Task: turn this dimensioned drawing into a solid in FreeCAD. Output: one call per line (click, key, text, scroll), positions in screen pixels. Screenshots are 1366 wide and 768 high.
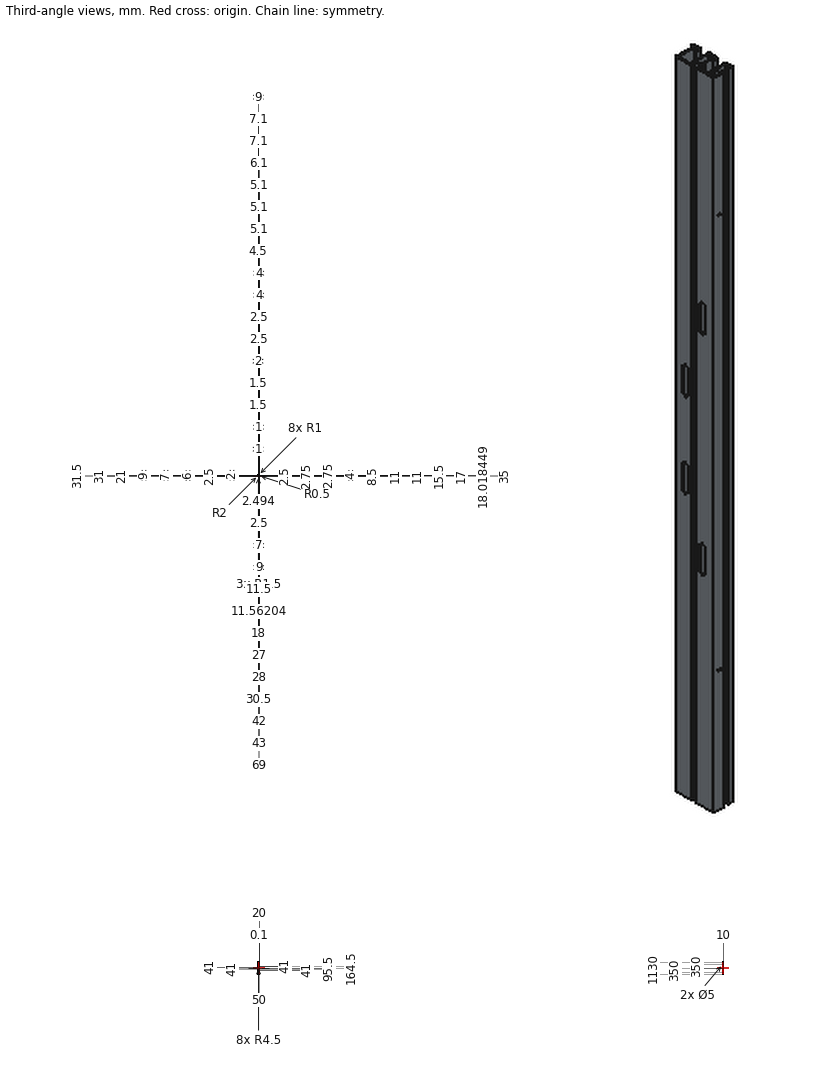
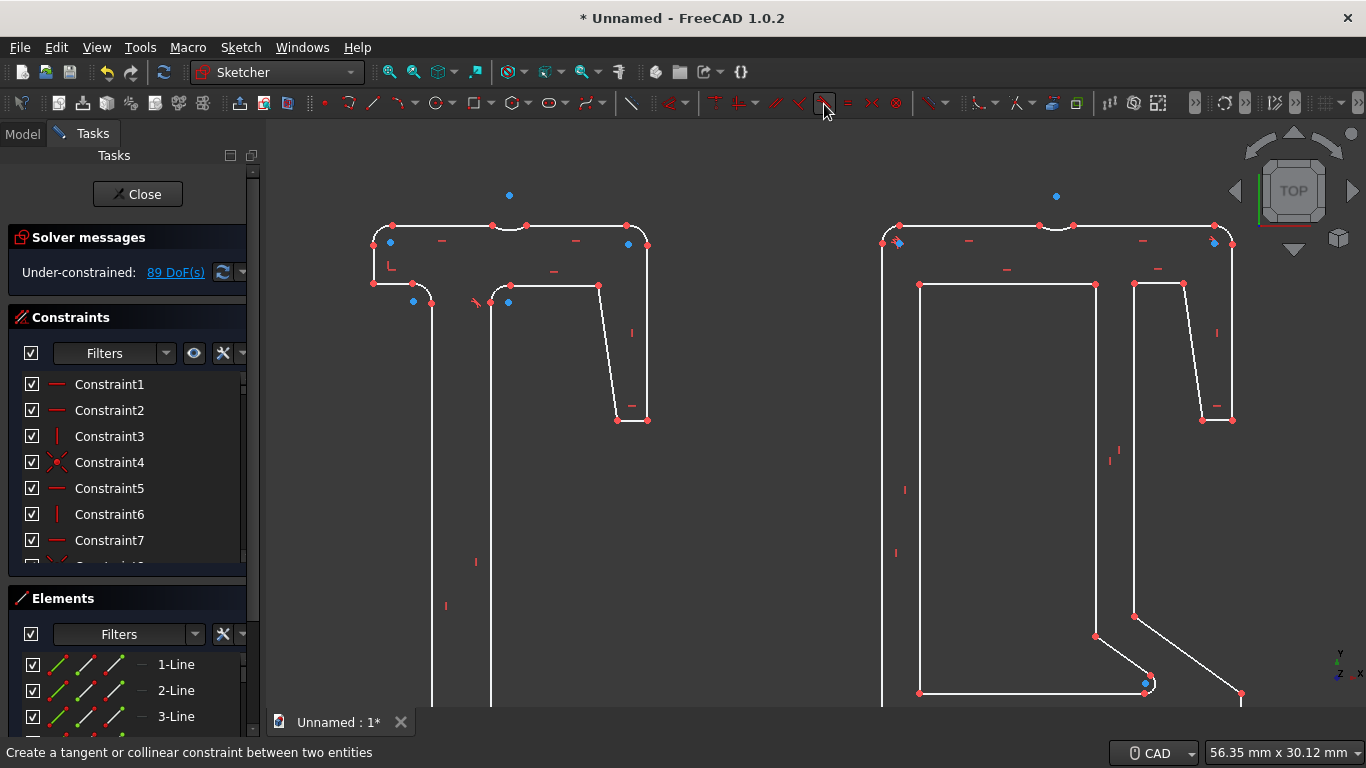
click(537, 286)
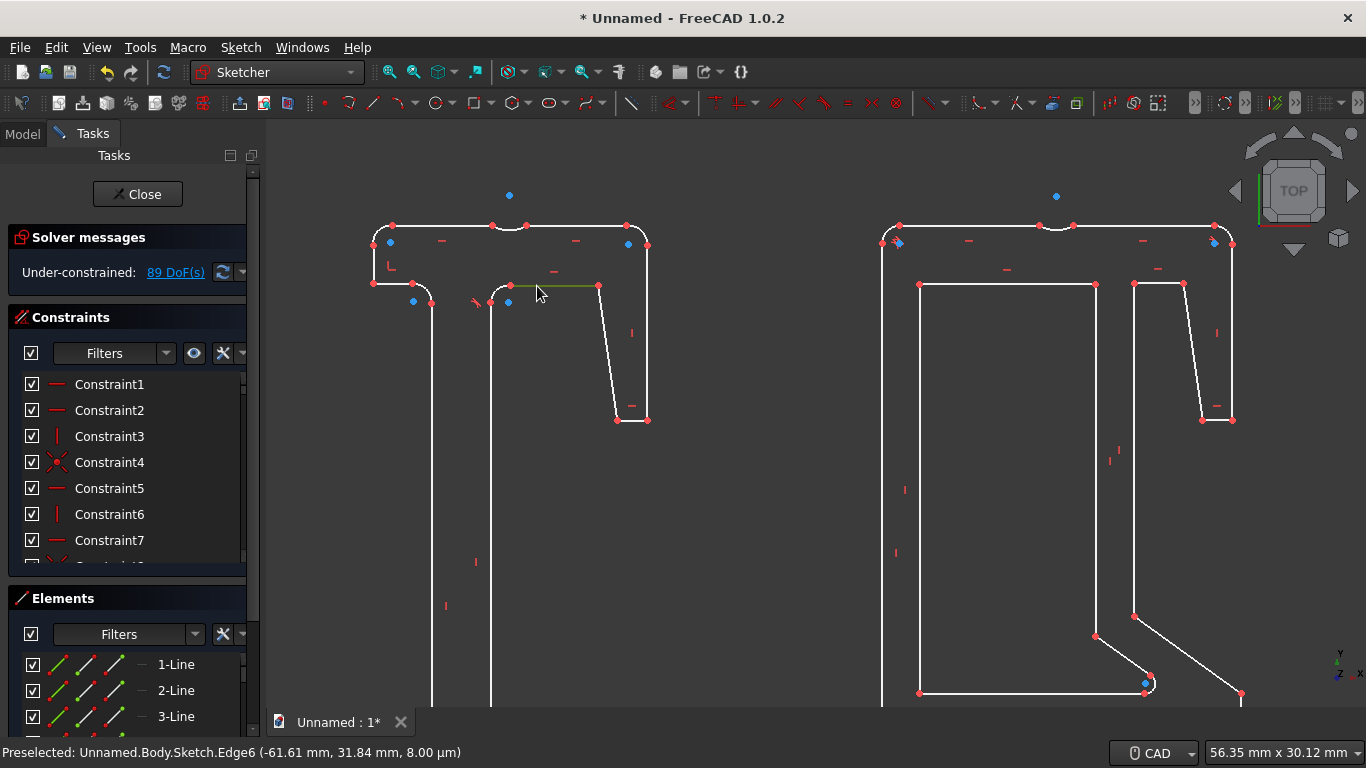
click(497, 290)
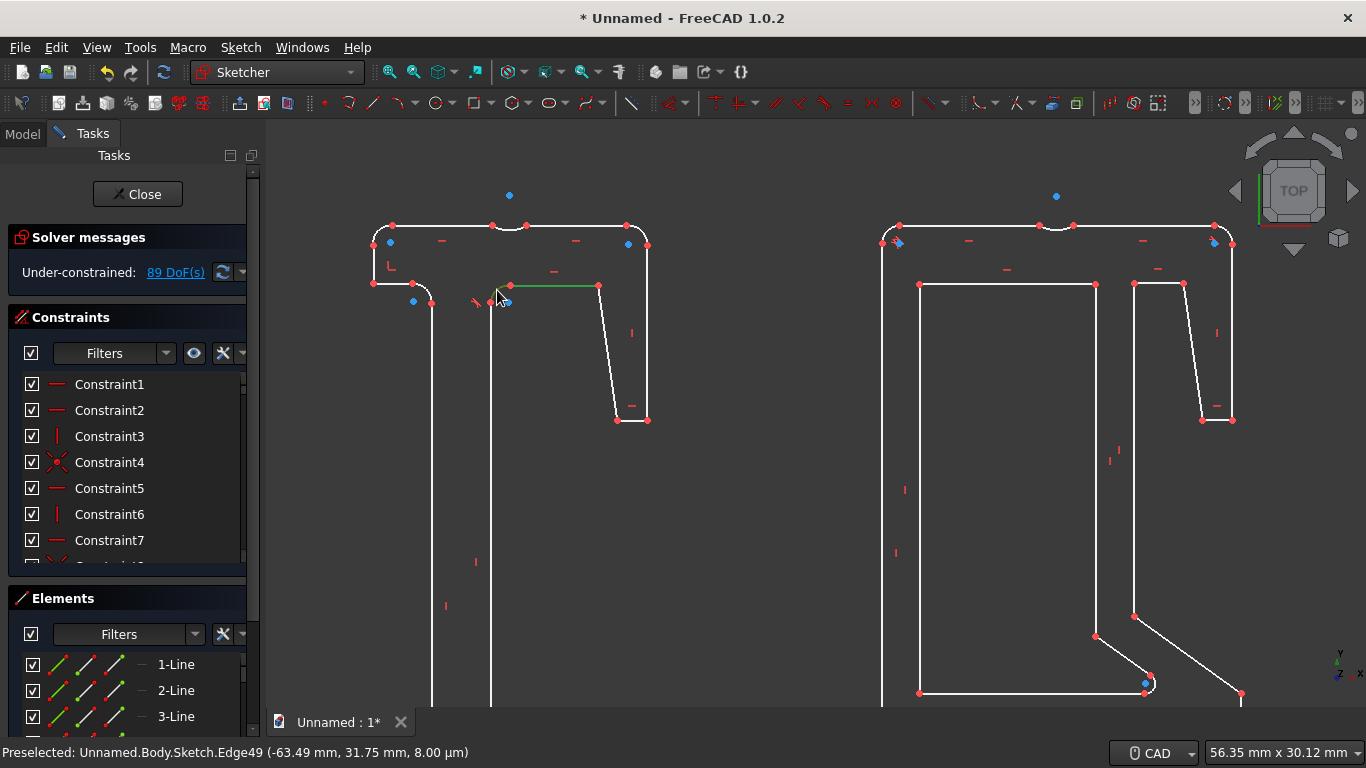
click(824, 104)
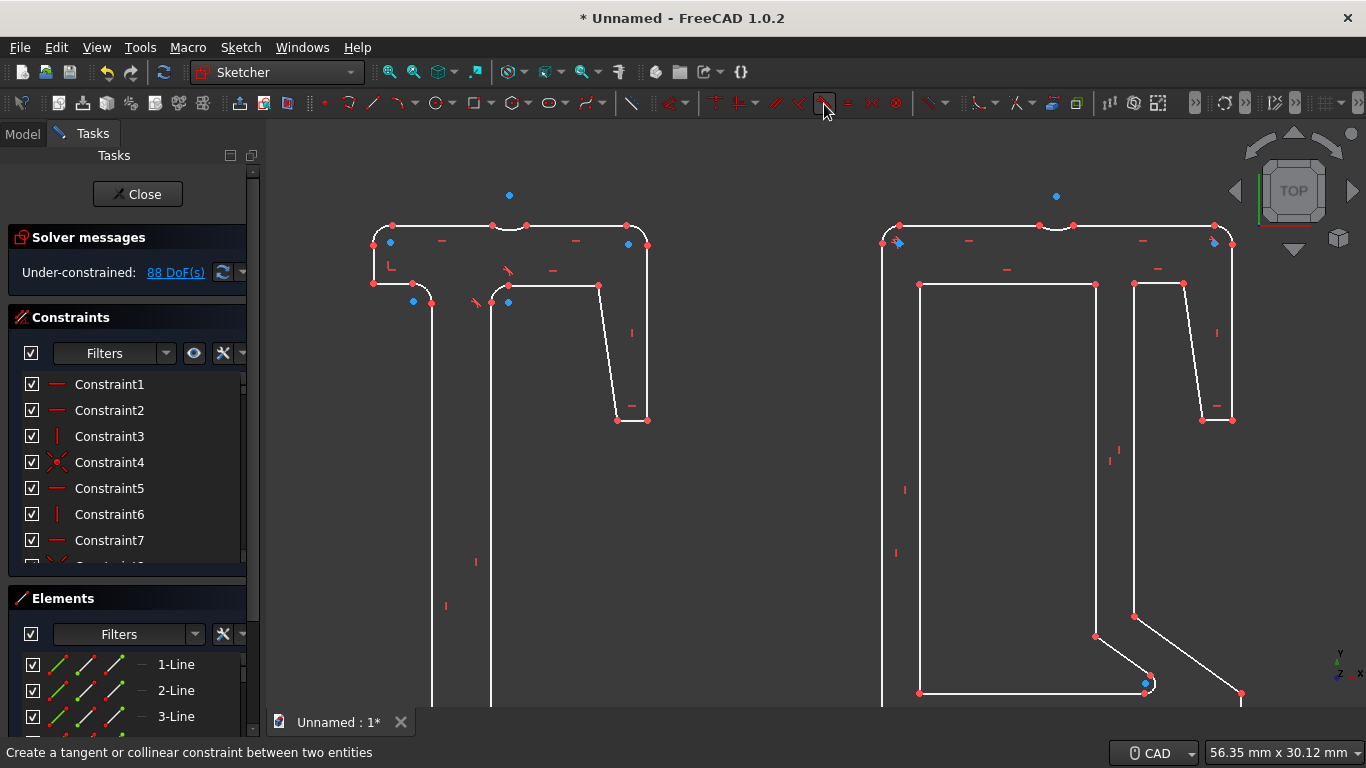
click(647, 368)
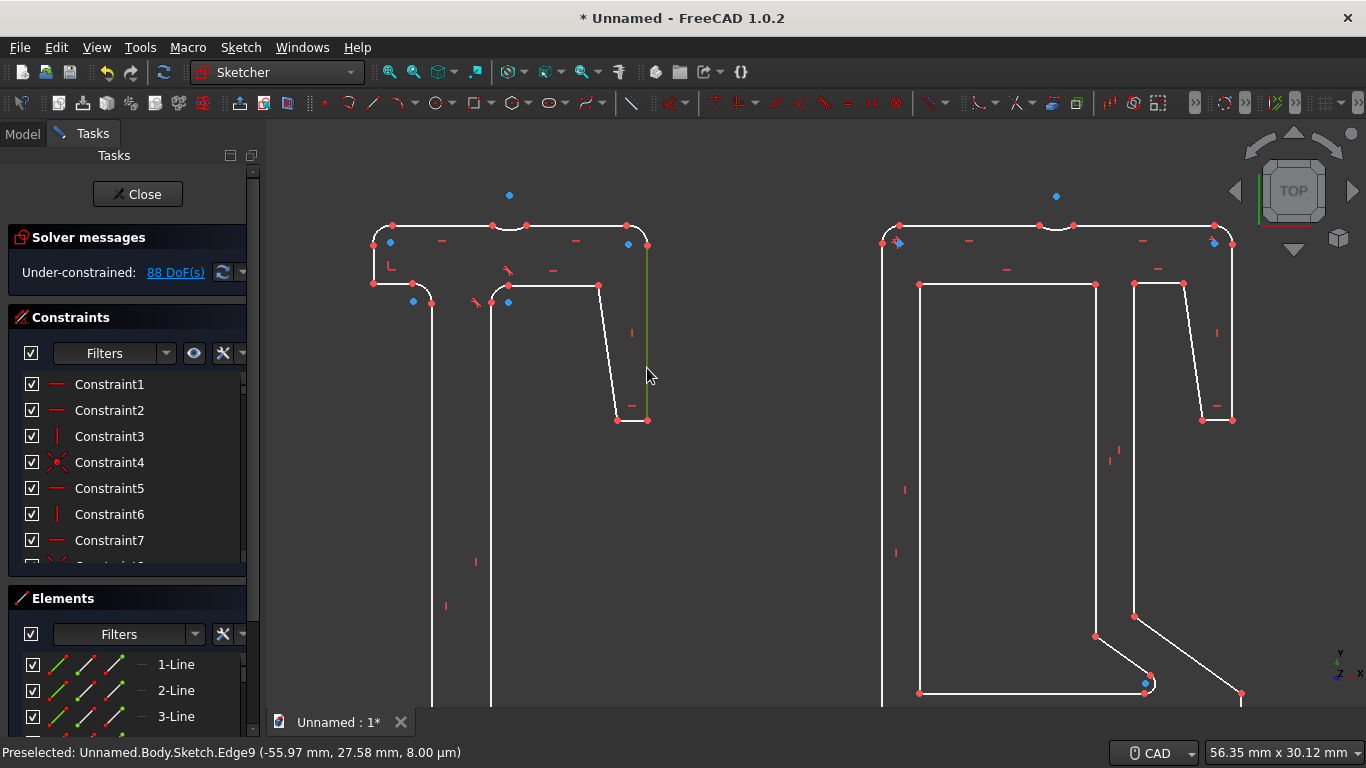
scroll(645, 236, up, 2)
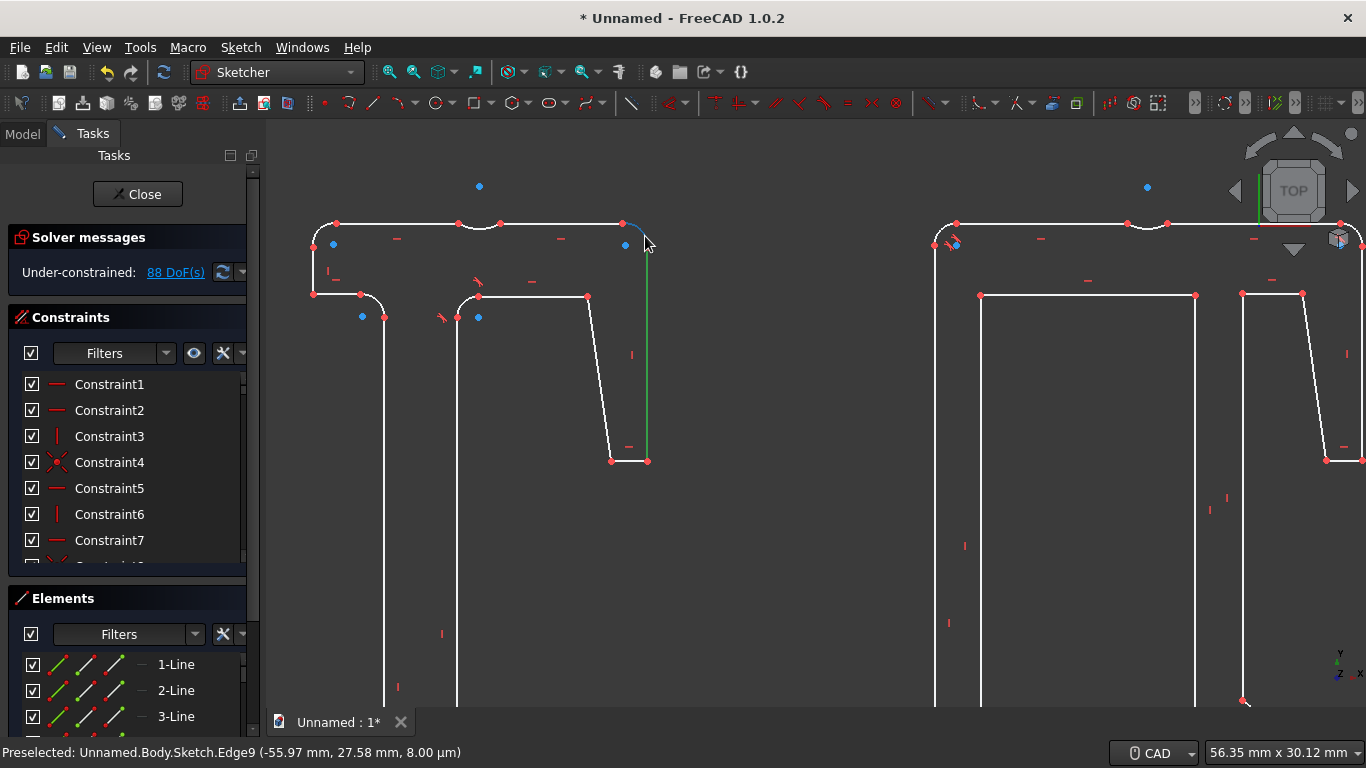
click(645, 236)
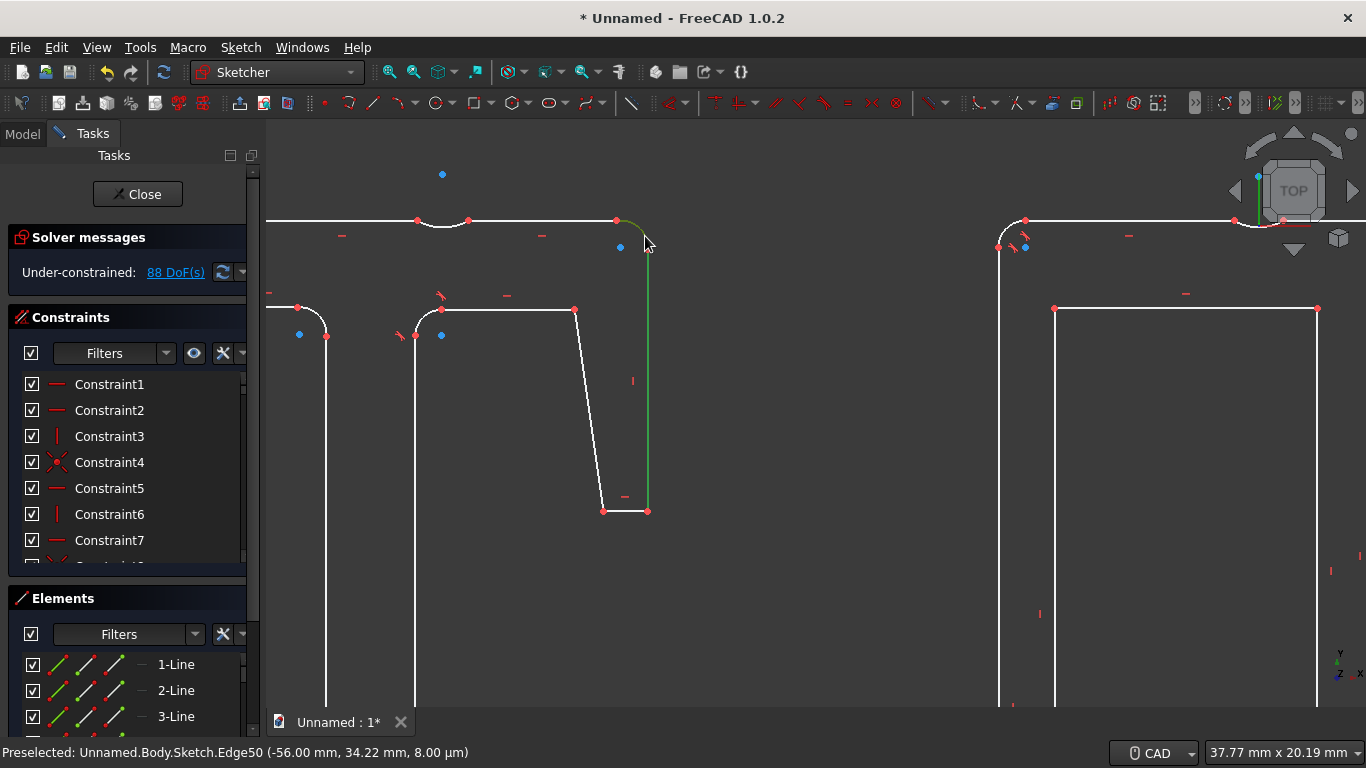
click(824, 104)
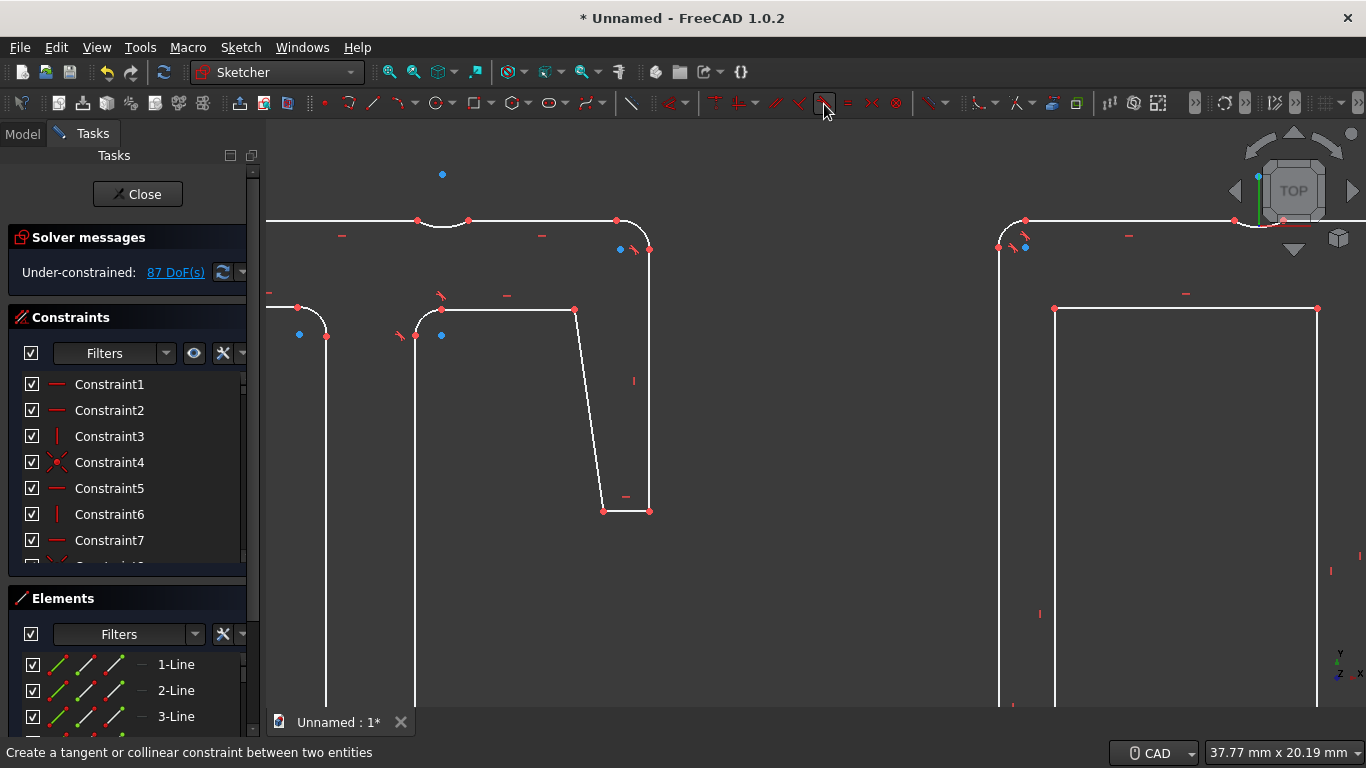
click(572, 221)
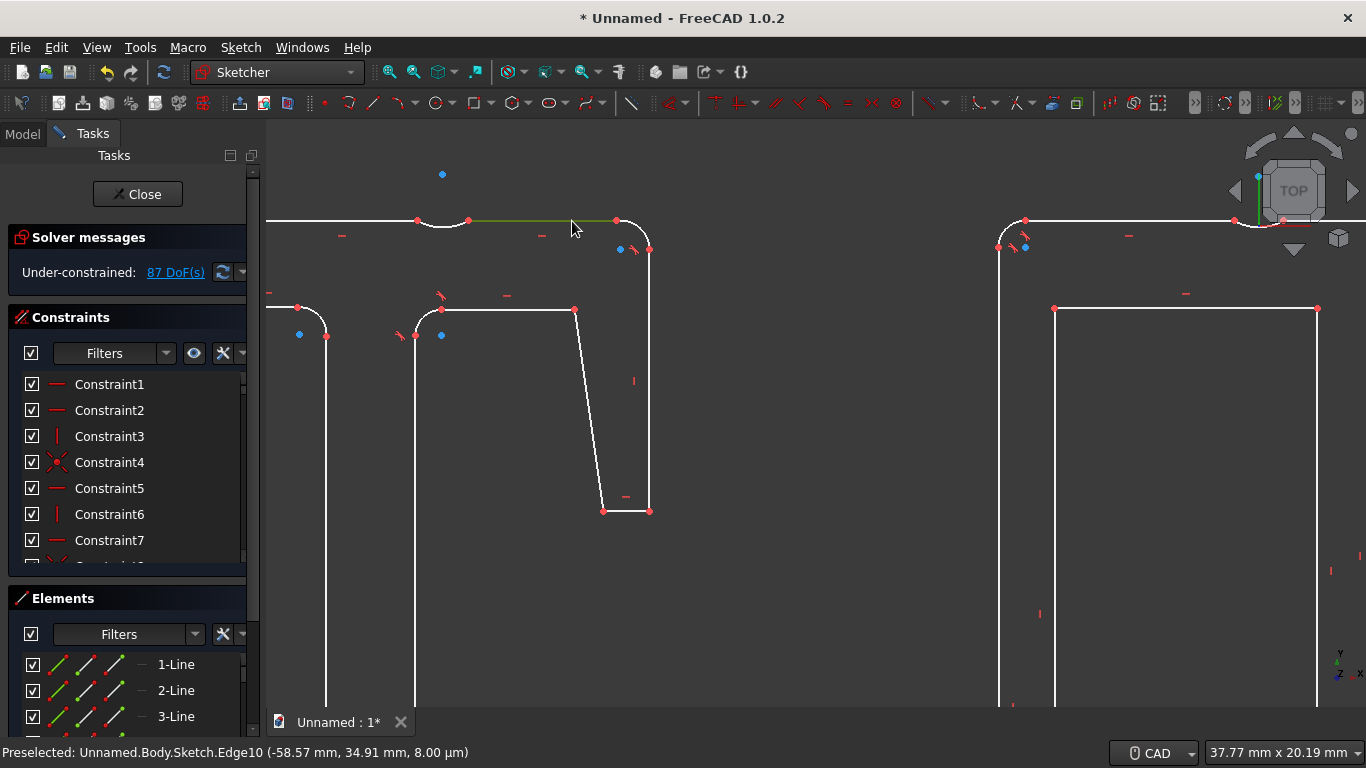
click(646, 235)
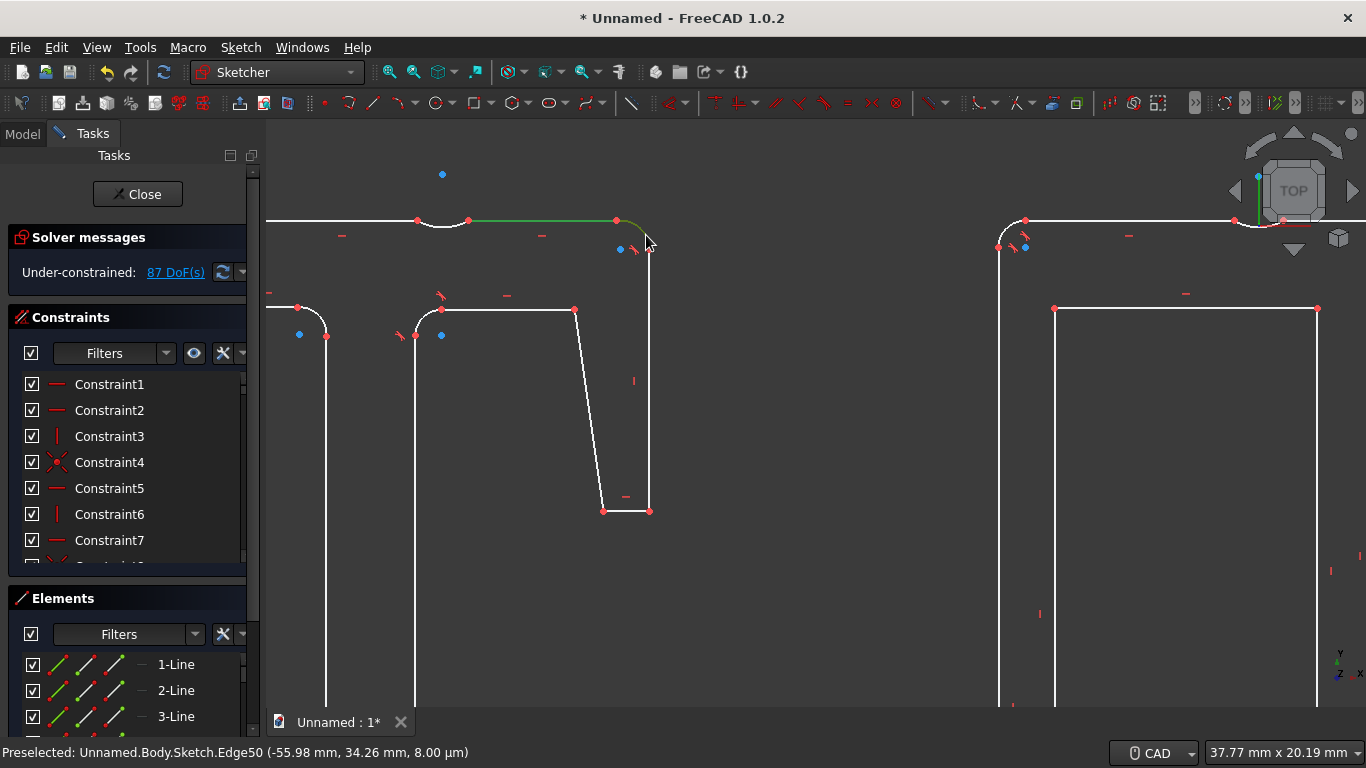
click(824, 104)